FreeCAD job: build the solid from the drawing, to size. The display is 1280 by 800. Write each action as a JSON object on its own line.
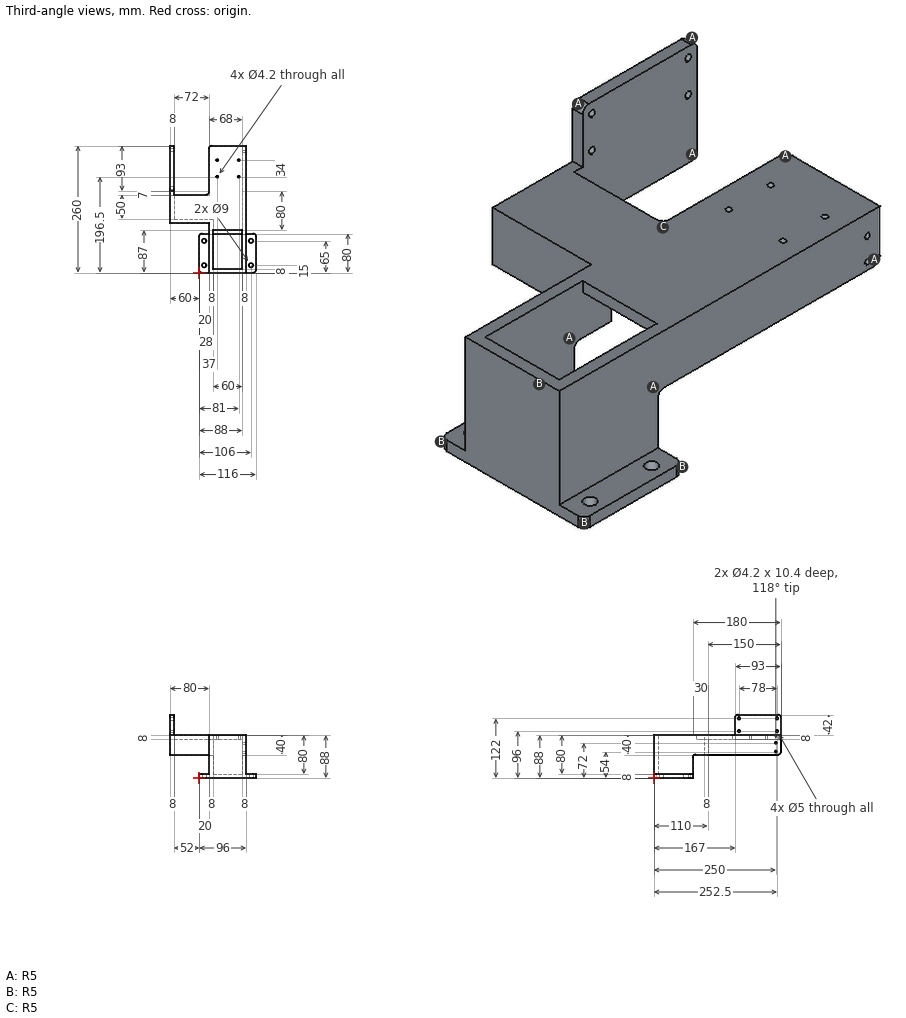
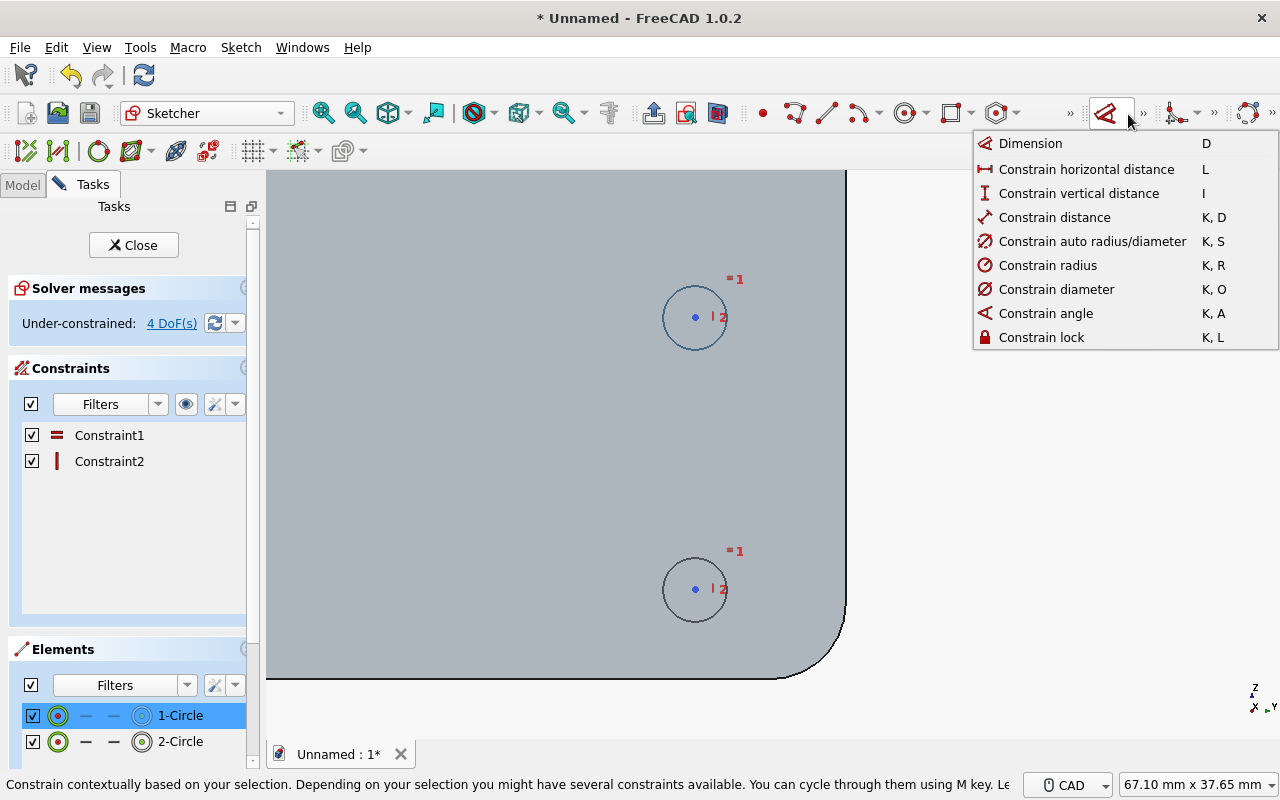
{"action": "left_click", "coordinate": [1126, 289]}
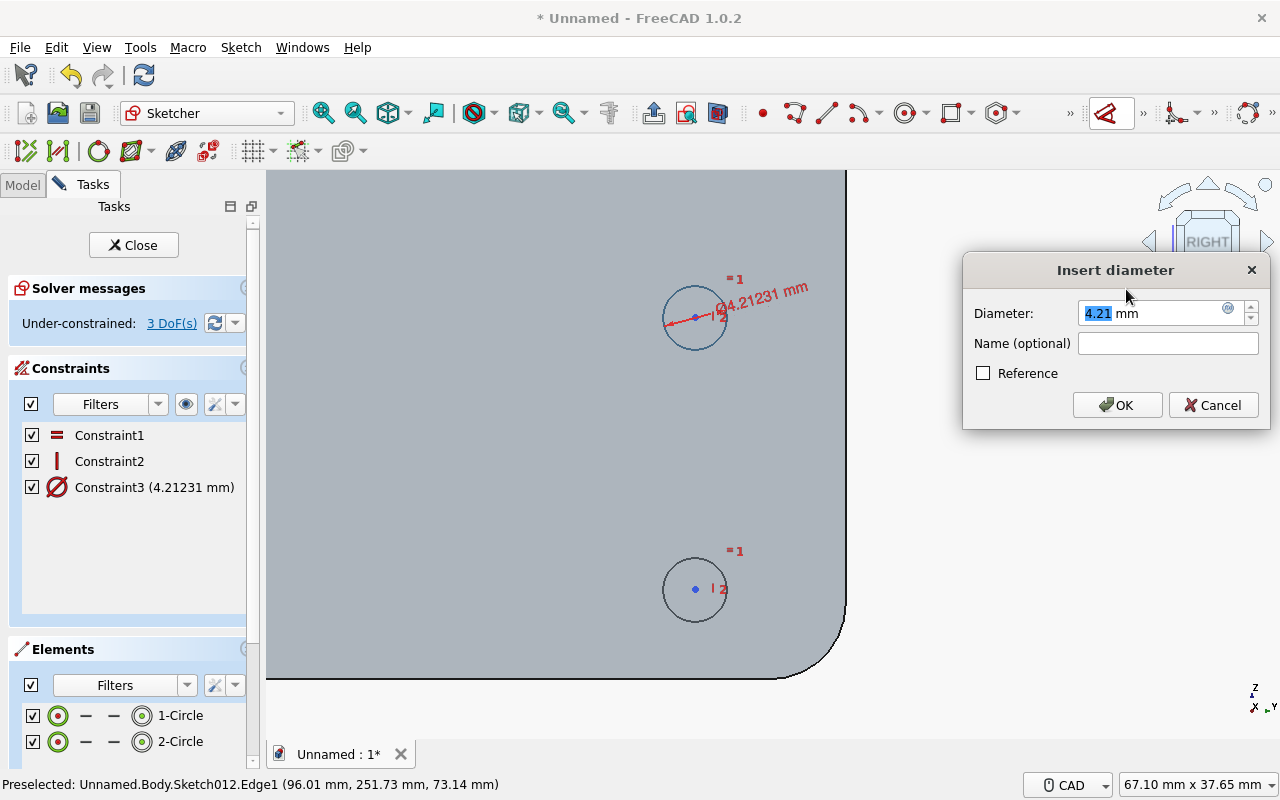
{"action": "type", "text": "4.2"}
{"action": "key", "text": "Return"}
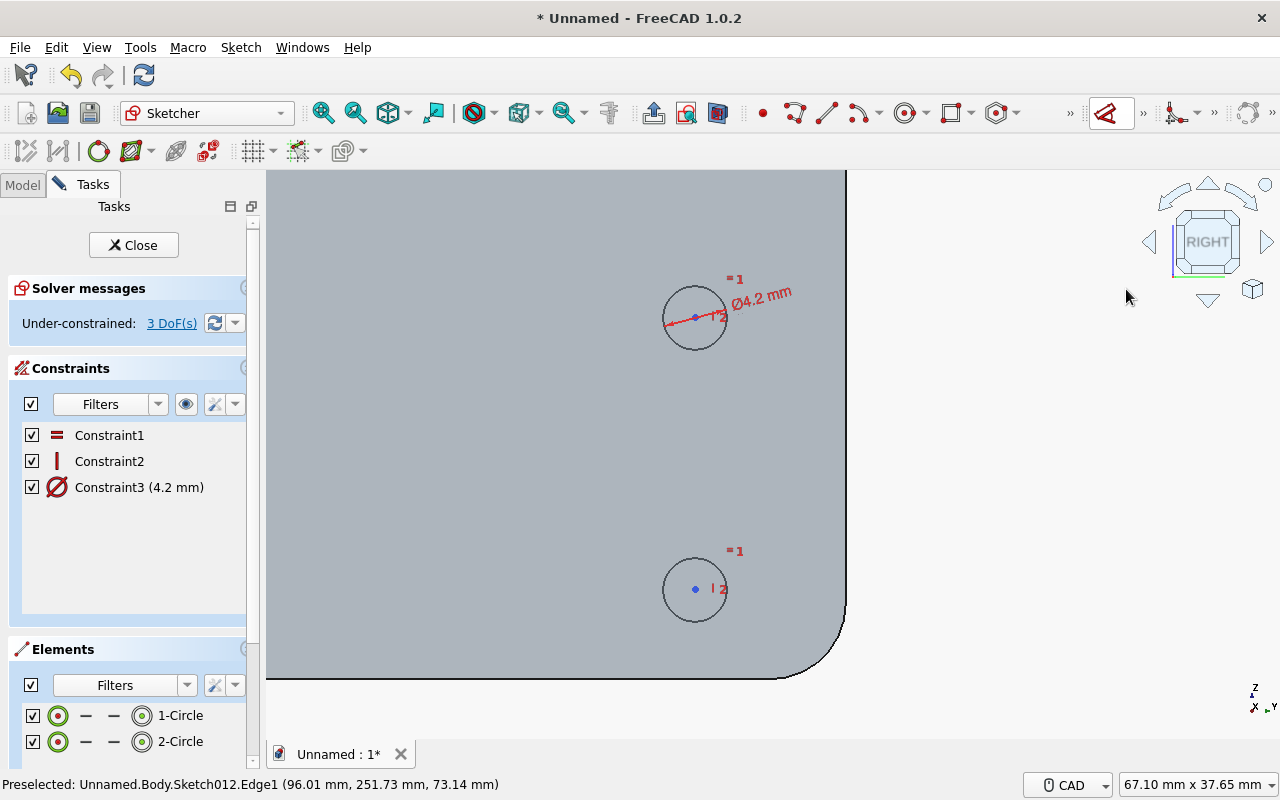
{"action": "left_click", "coordinate": [695, 318]}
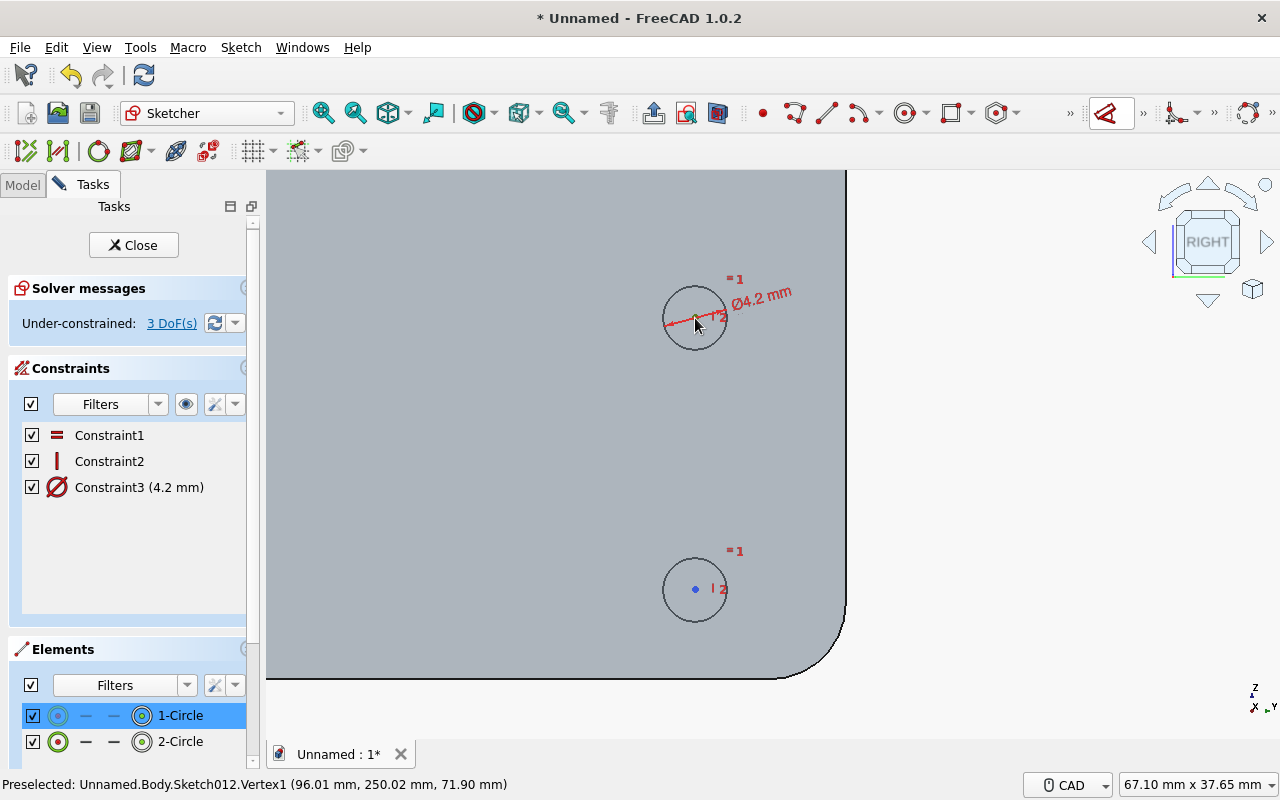
{"action": "left_click", "coordinate": [1128, 114]}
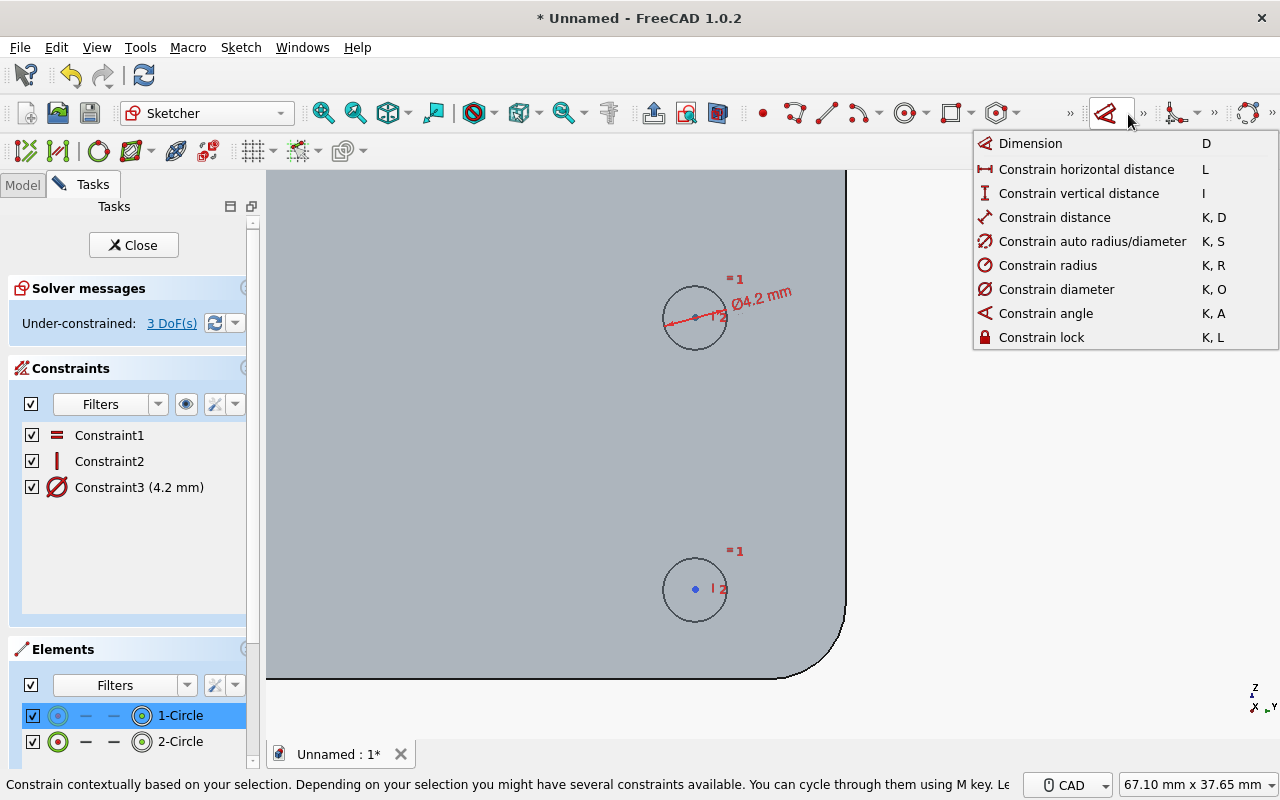
{"action": "left_click", "coordinate": [1126, 193]}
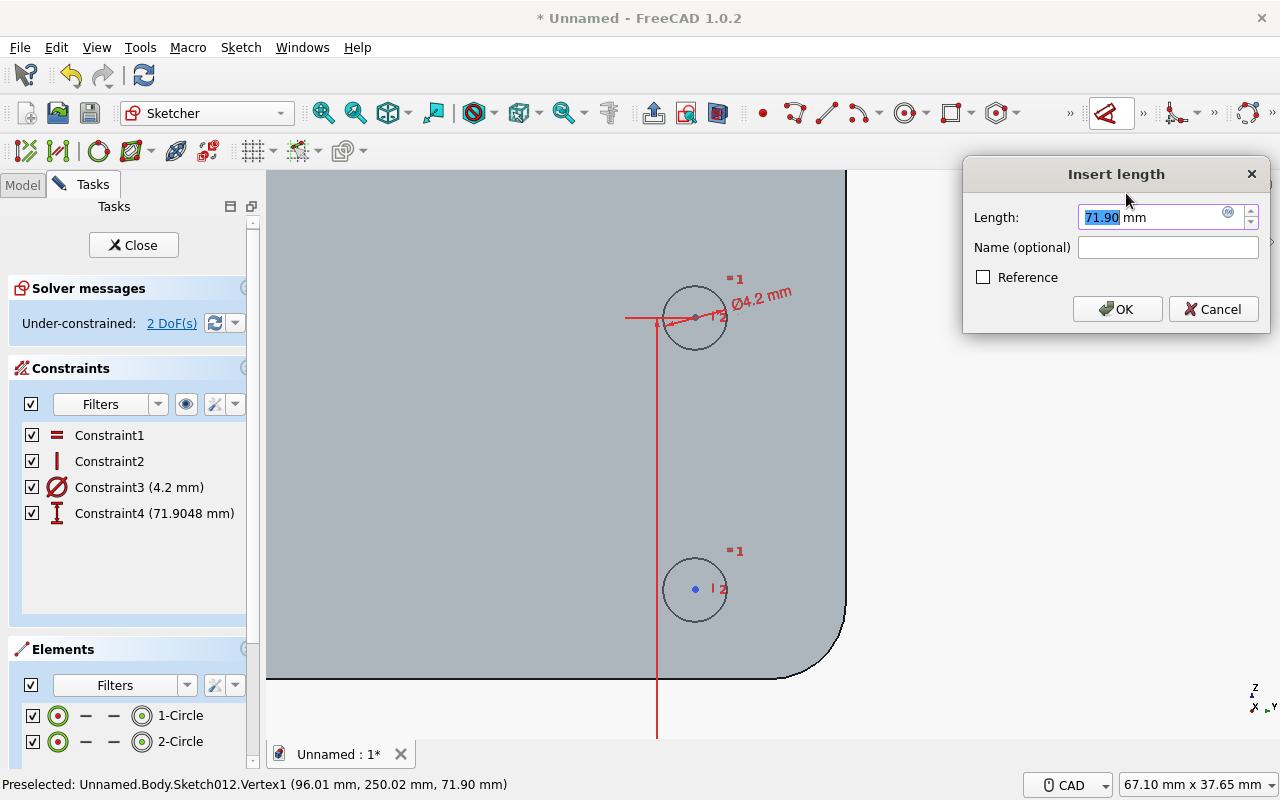
{"action": "type", "text": "72"}
{"action": "key", "text": "Return"}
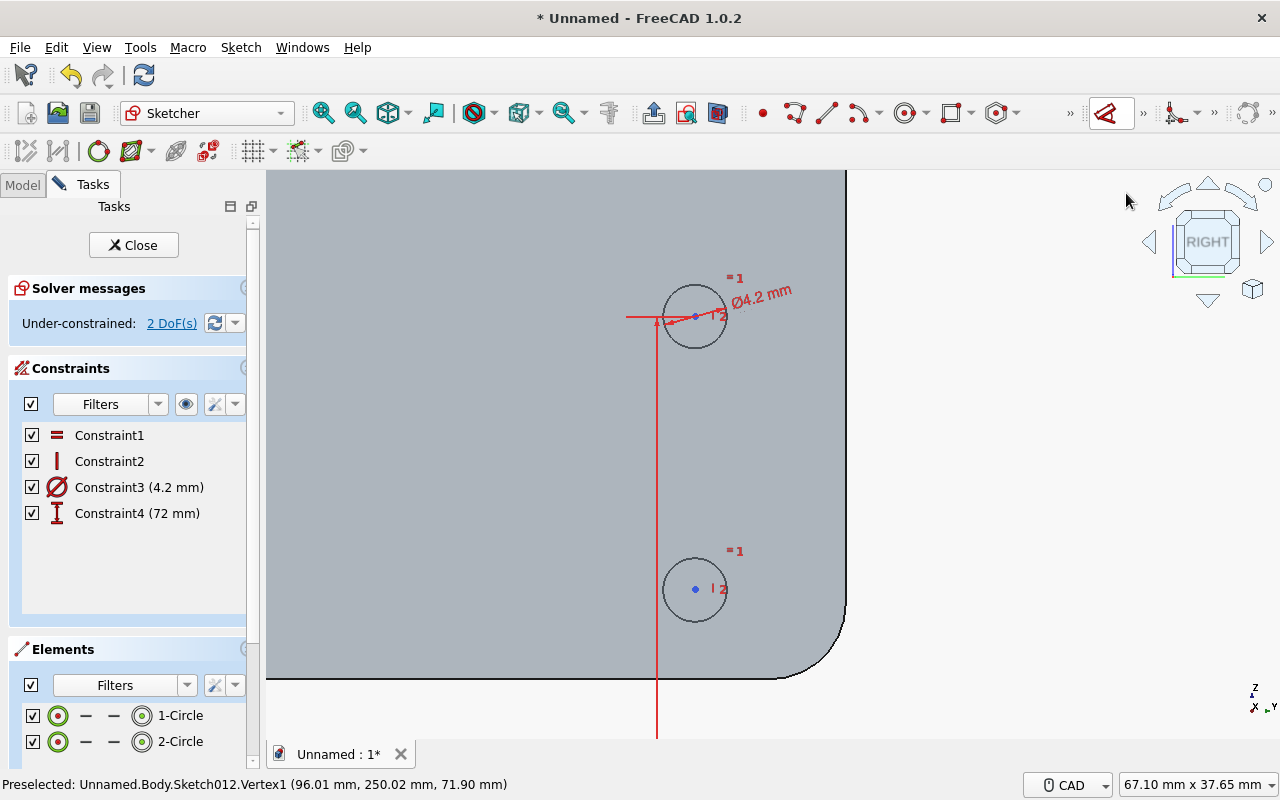
{"action": "left_click", "coordinate": [695, 590]}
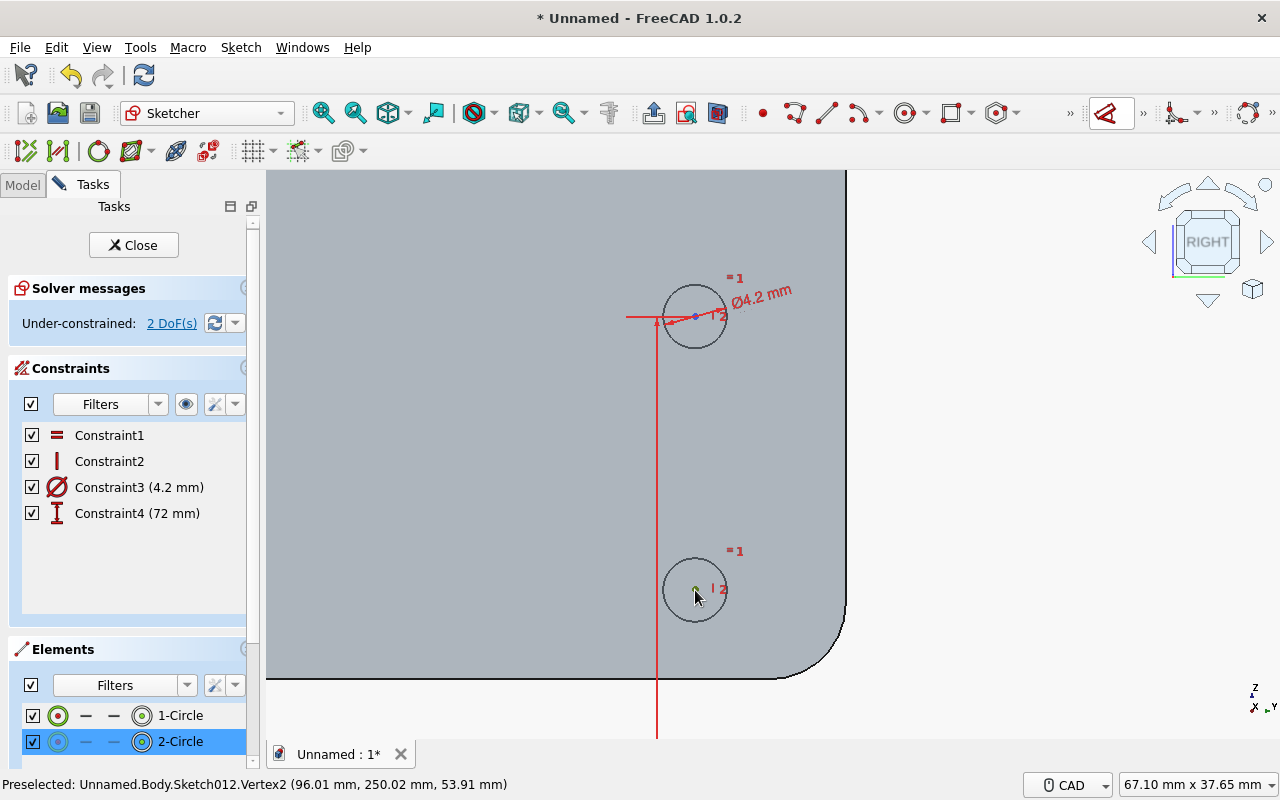
{"action": "left_click", "coordinate": [1128, 114]}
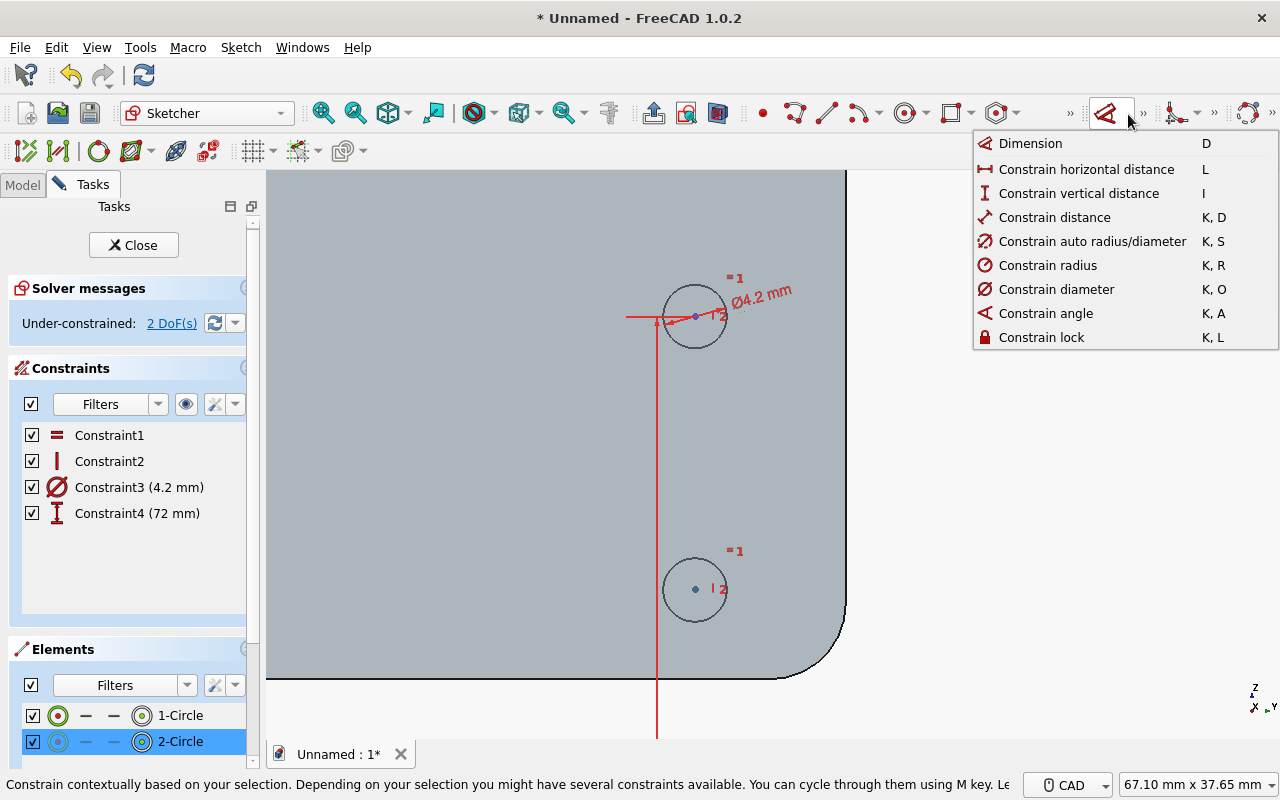
{"action": "left_click", "coordinate": [1126, 193]}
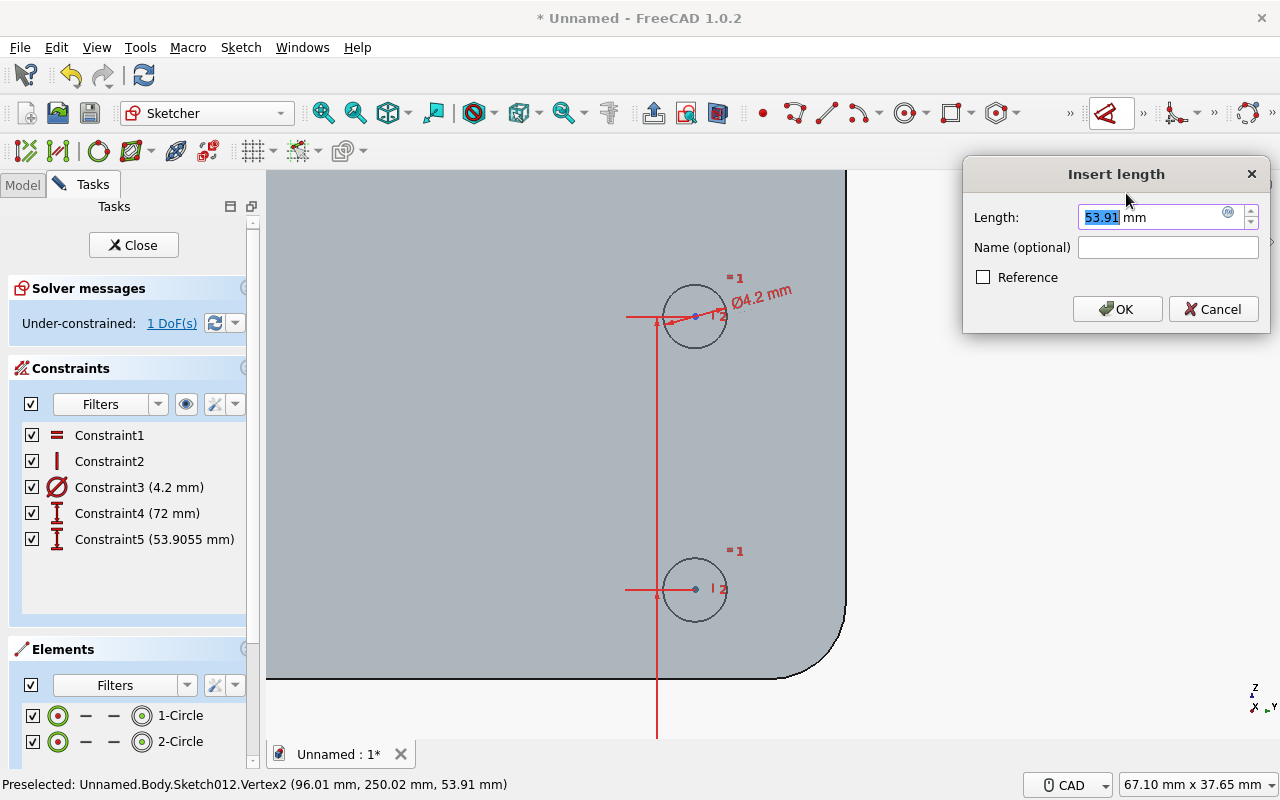
{"action": "type", "text": "54"}
{"action": "key", "text": "Return"}